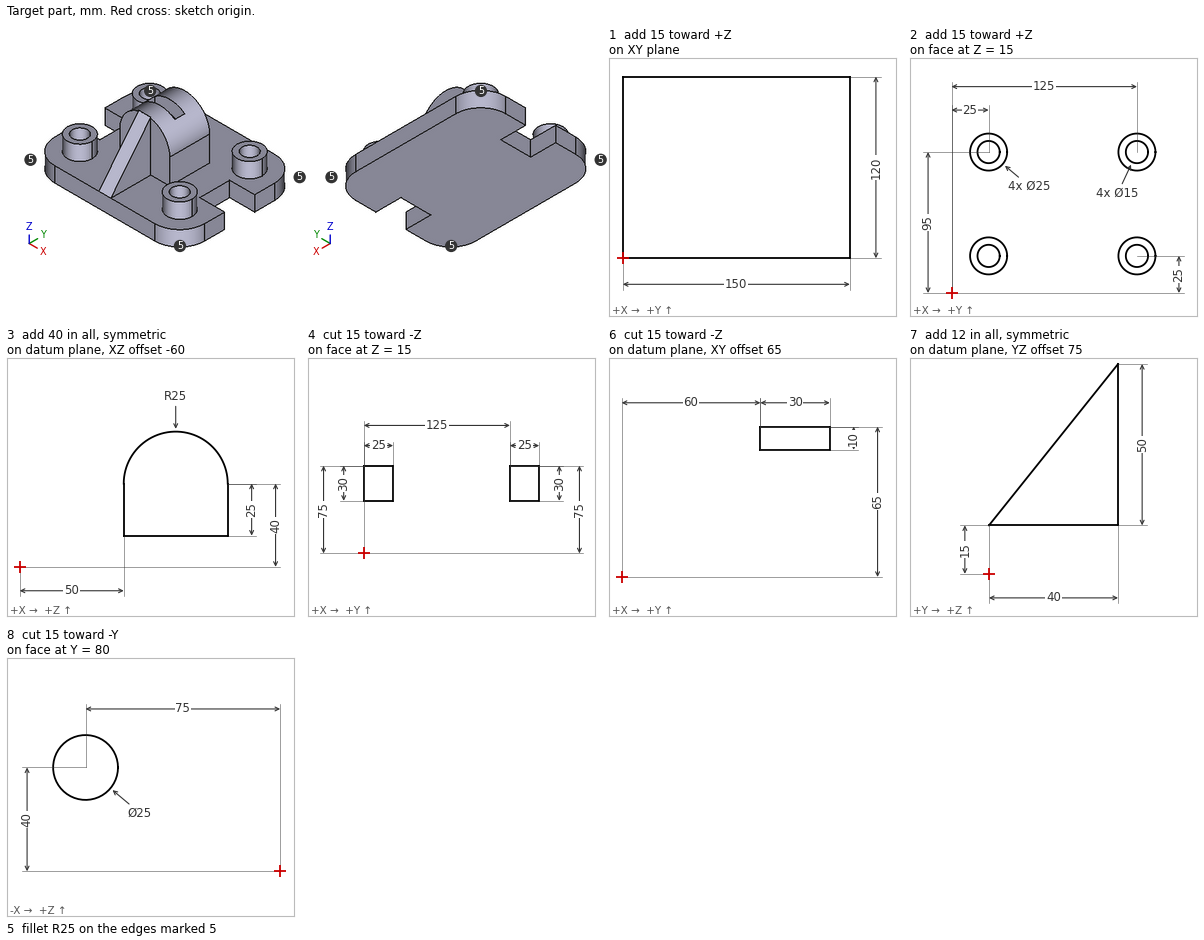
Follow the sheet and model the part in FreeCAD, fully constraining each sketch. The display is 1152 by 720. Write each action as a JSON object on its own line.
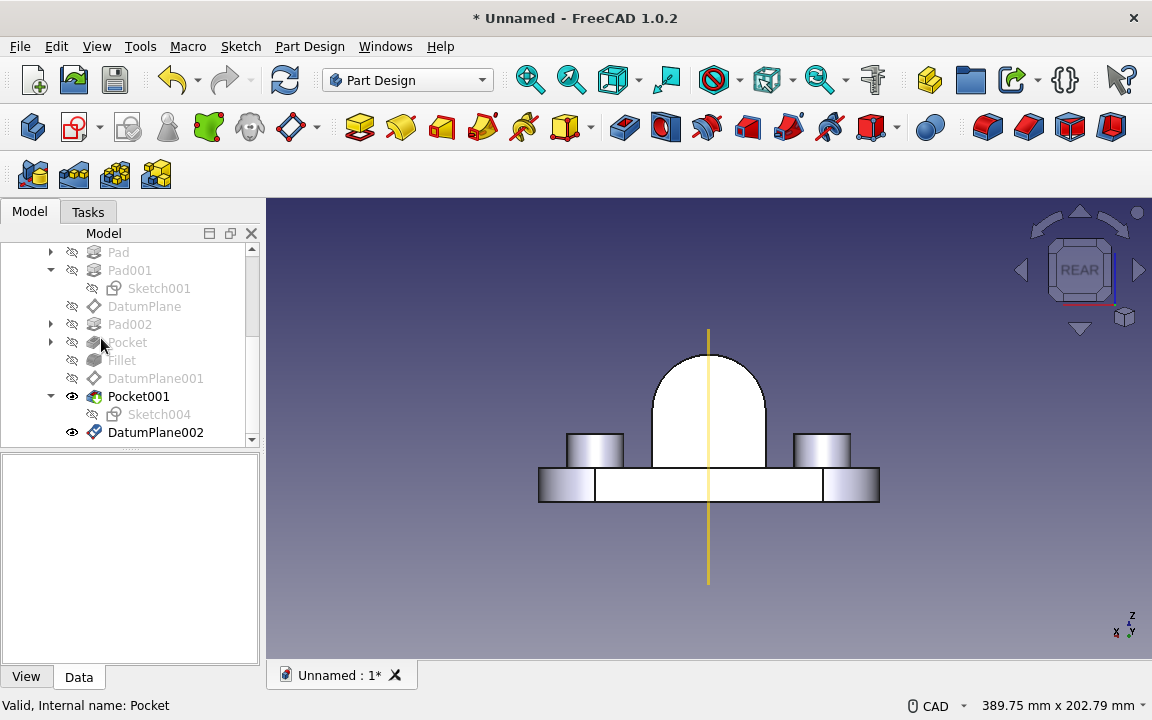
{"action": "left_click", "coordinate": [117, 432]}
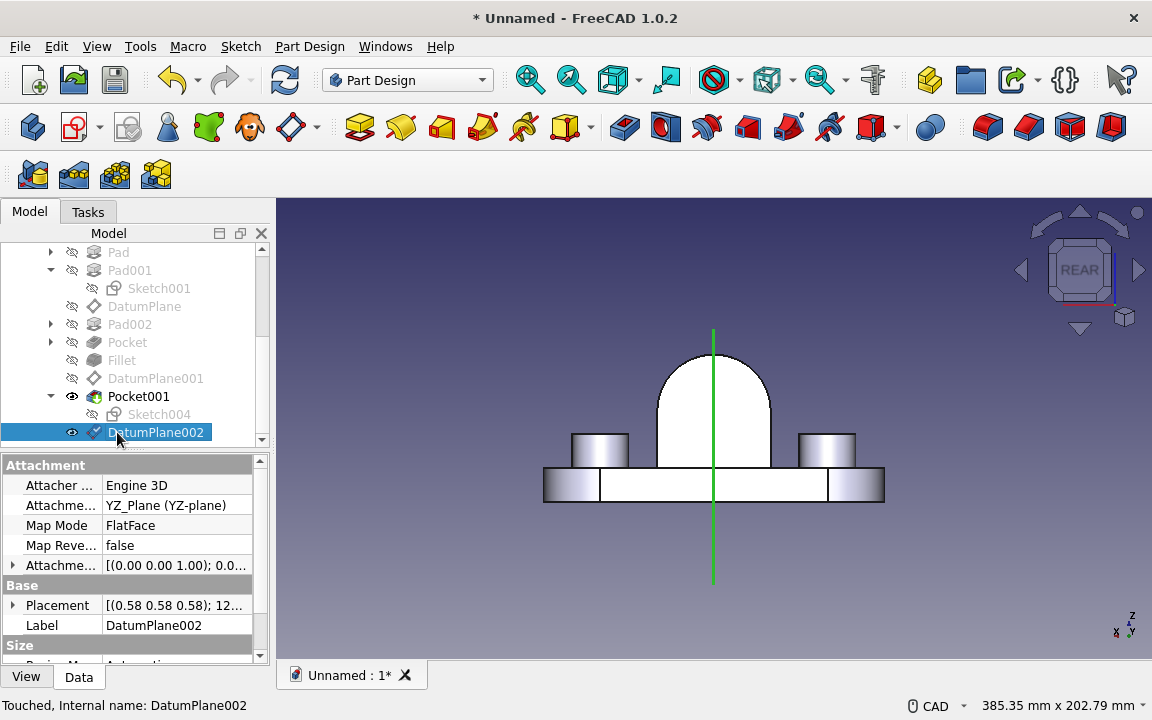
{"action": "left_click", "coordinate": [74, 128]}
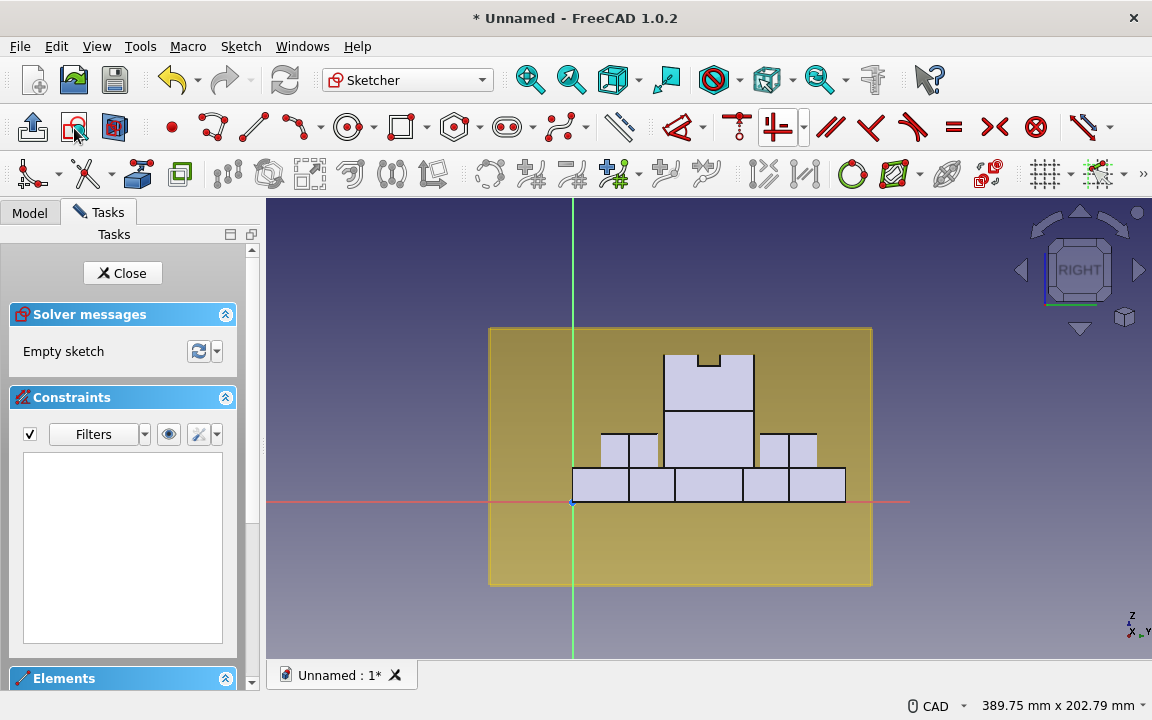
{"action": "key", "text": "q s"}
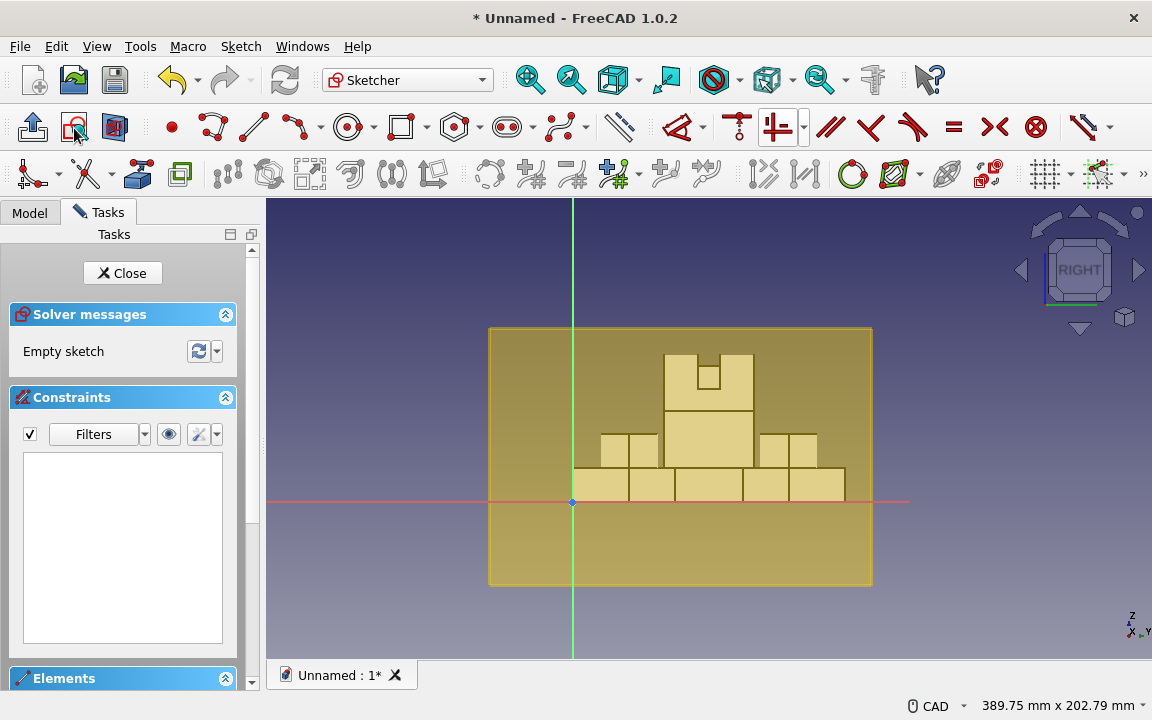
{"action": "scroll", "coordinate": [591, 428], "scroll_direction": "up", "scroll_amount": 3}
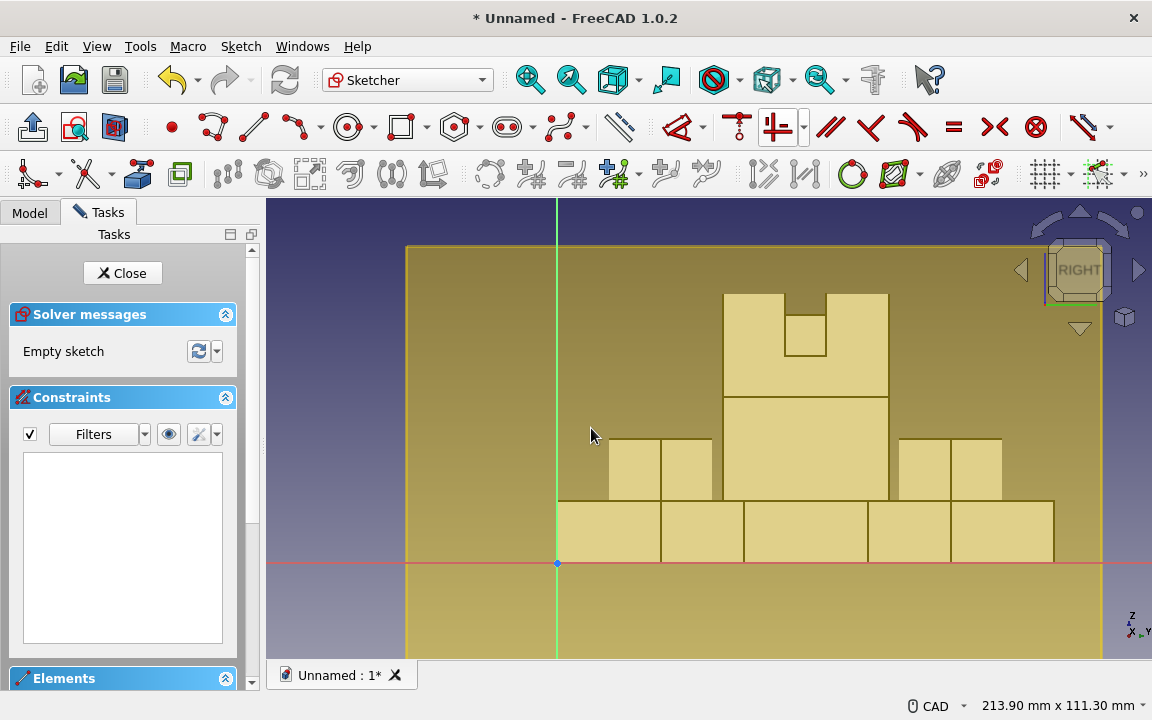
{"action": "left_click", "coordinate": [213, 128]}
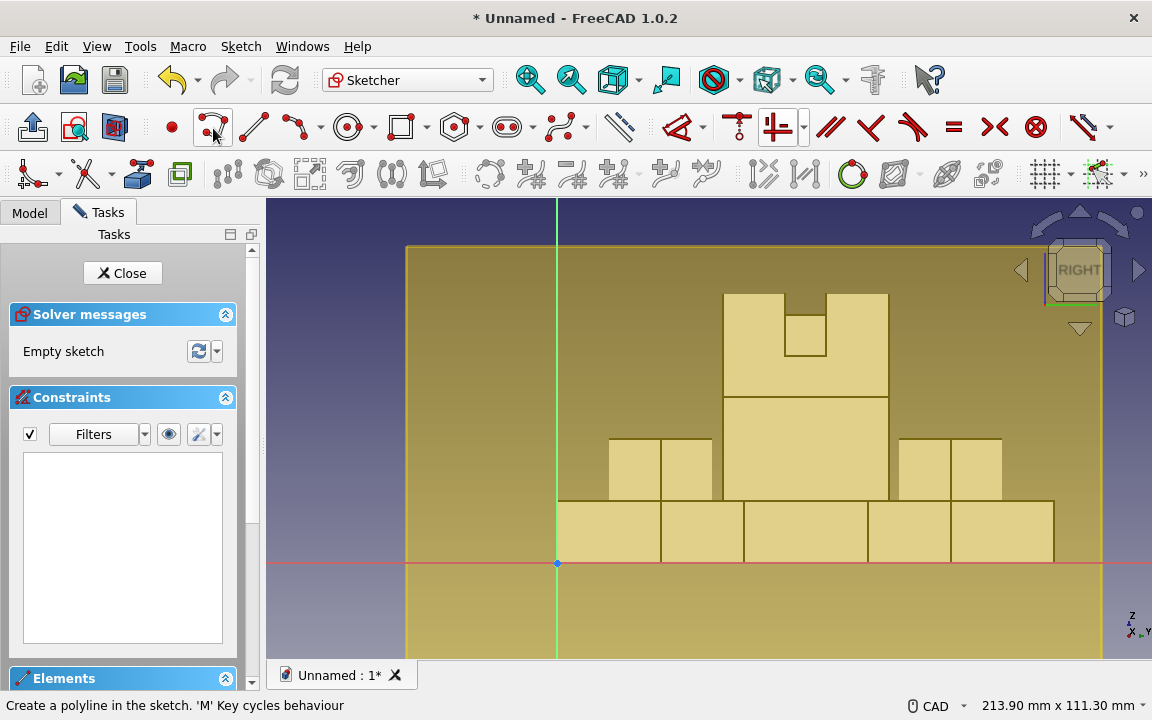
{"action": "left_click", "coordinate": [557, 501]}
{"action": "left_click", "coordinate": [723, 501]}
{"action": "left_click", "coordinate": [723, 294]}
{"action": "left_click", "coordinate": [557, 502]}
{"action": "key", "text": "Escape"}
{"action": "key", "text": "Escape"}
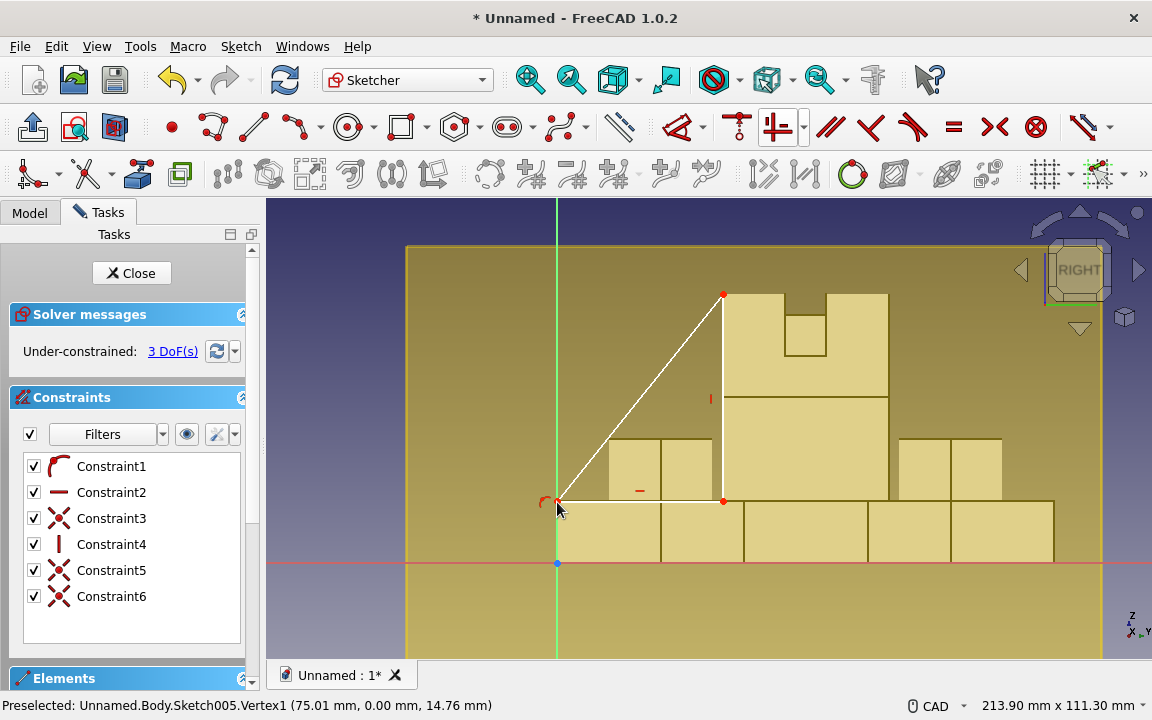
{"action": "left_click", "coordinate": [676, 128]}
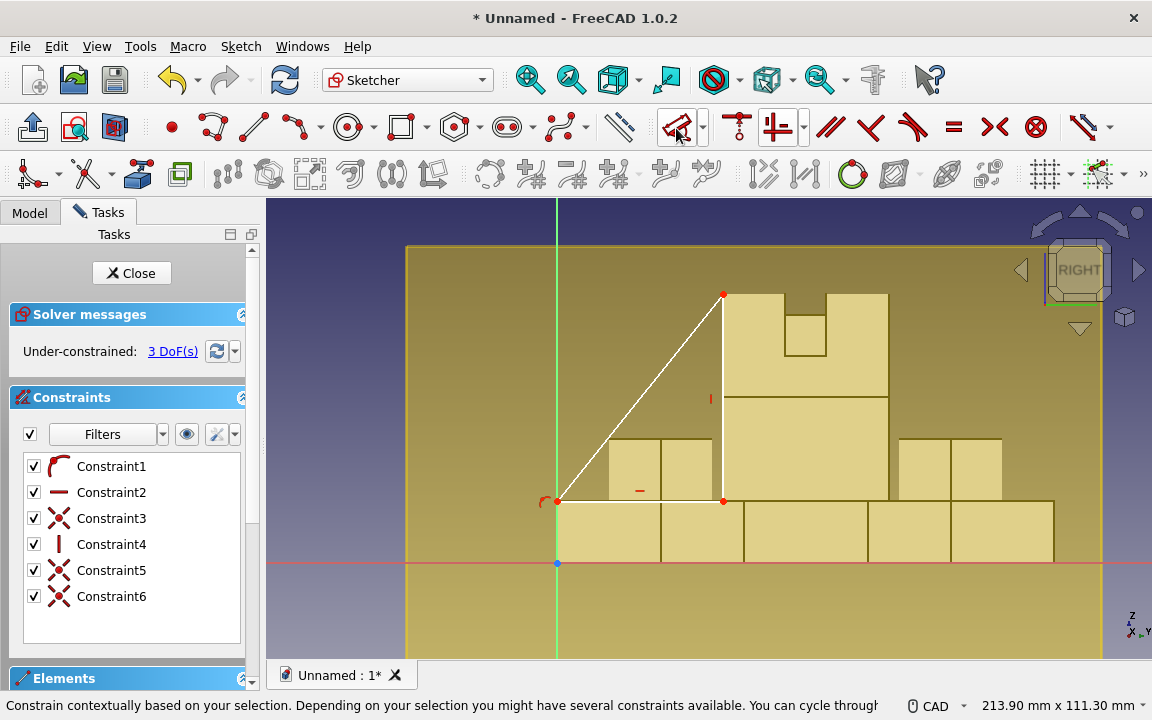
{"action": "left_click", "coordinate": [607, 502]}
{"action": "left_click", "coordinate": [640, 536]}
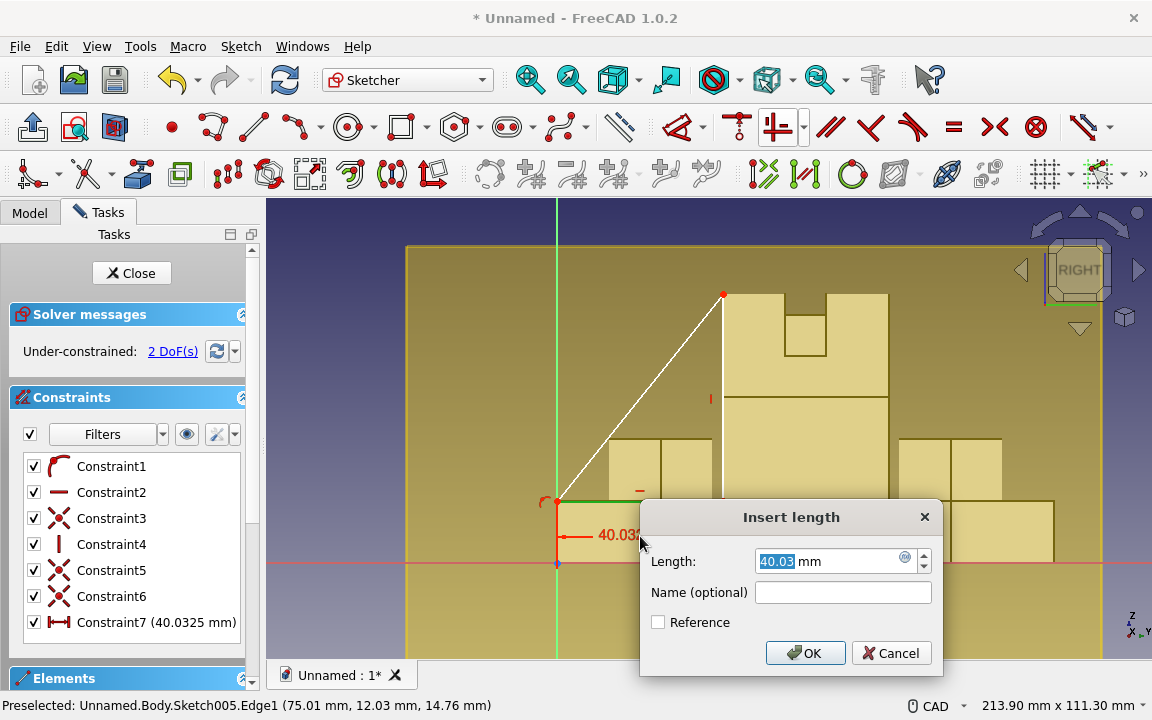
{"action": "type", "text": "40"}
{"action": "key", "text": "Return"}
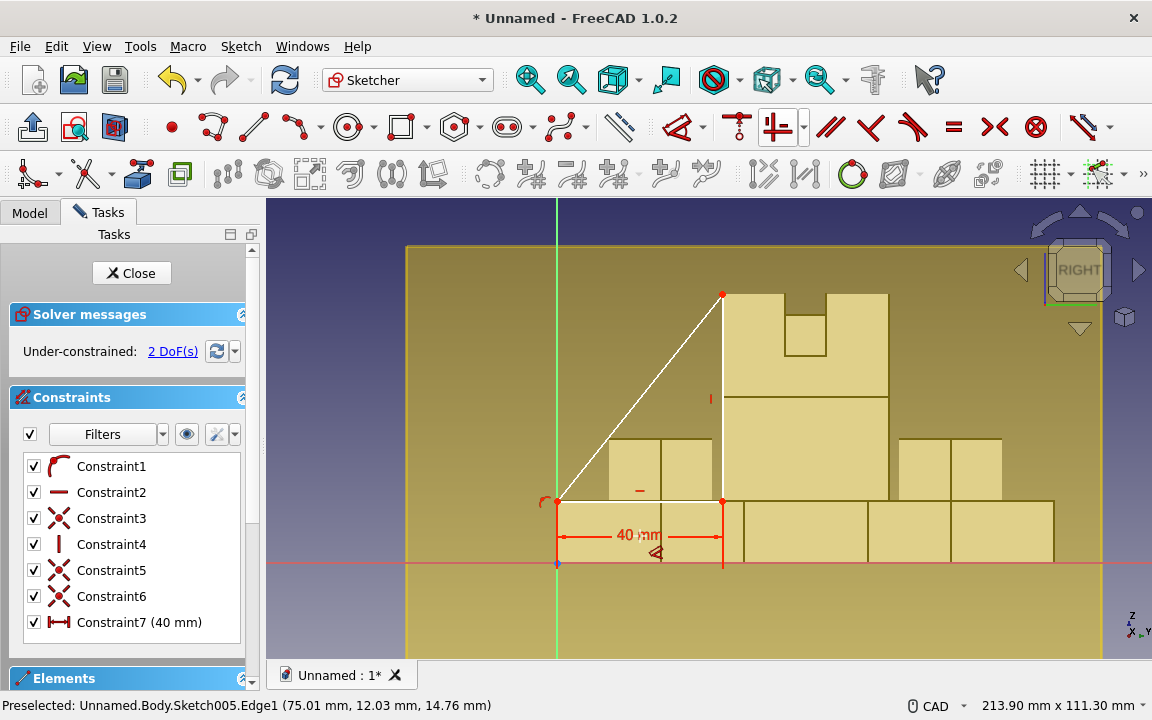
{"action": "left_click", "coordinate": [723, 440]}
{"action": "left_click", "coordinate": [757, 399]}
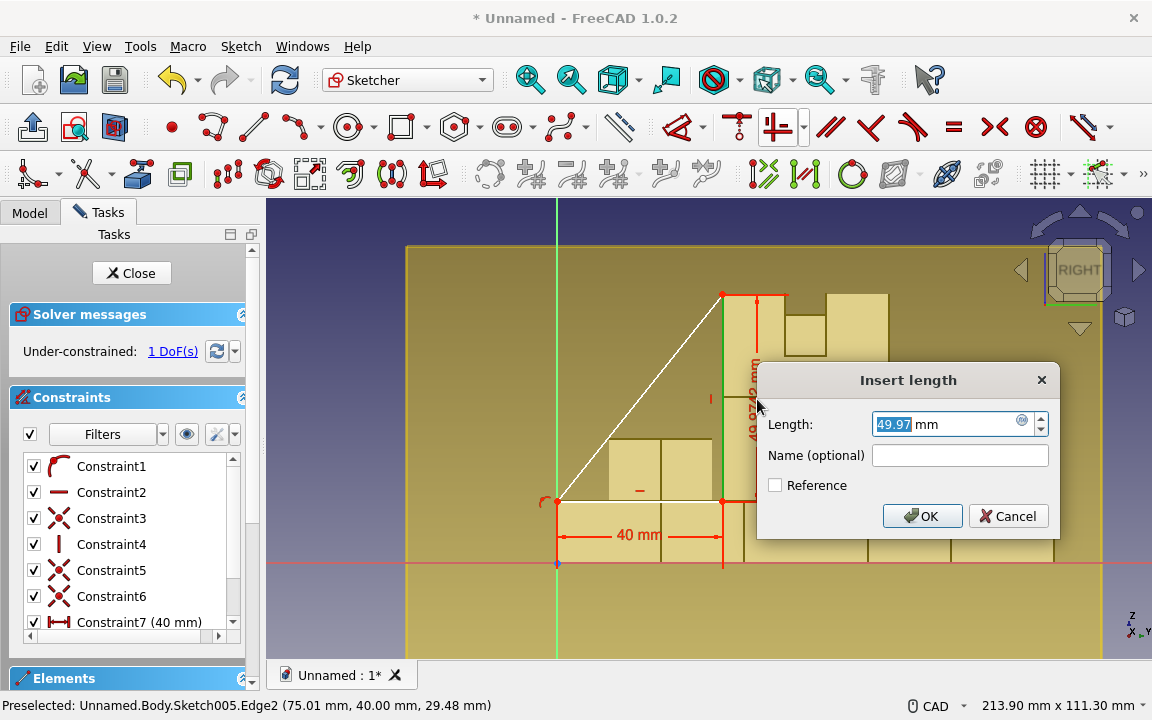
{"action": "type", "text": "50"}
{"action": "key", "text": "Return"}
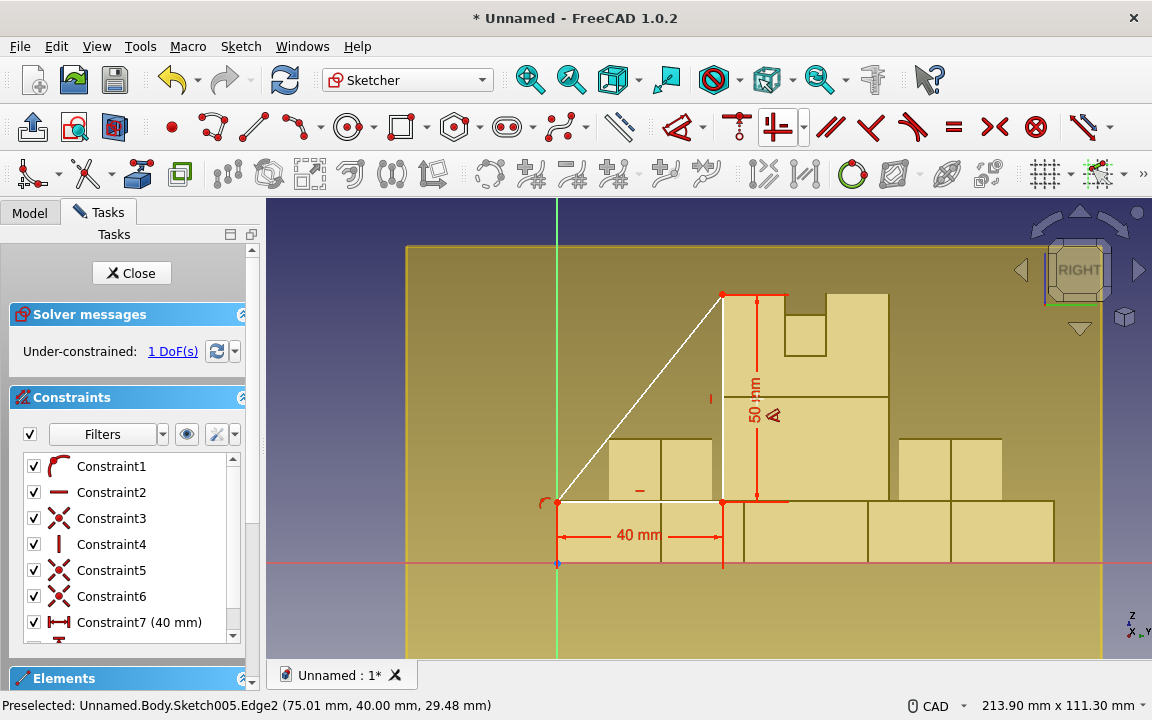
{"action": "left_click", "coordinate": [557, 502]}
{"action": "left_click", "coordinate": [523, 533]}